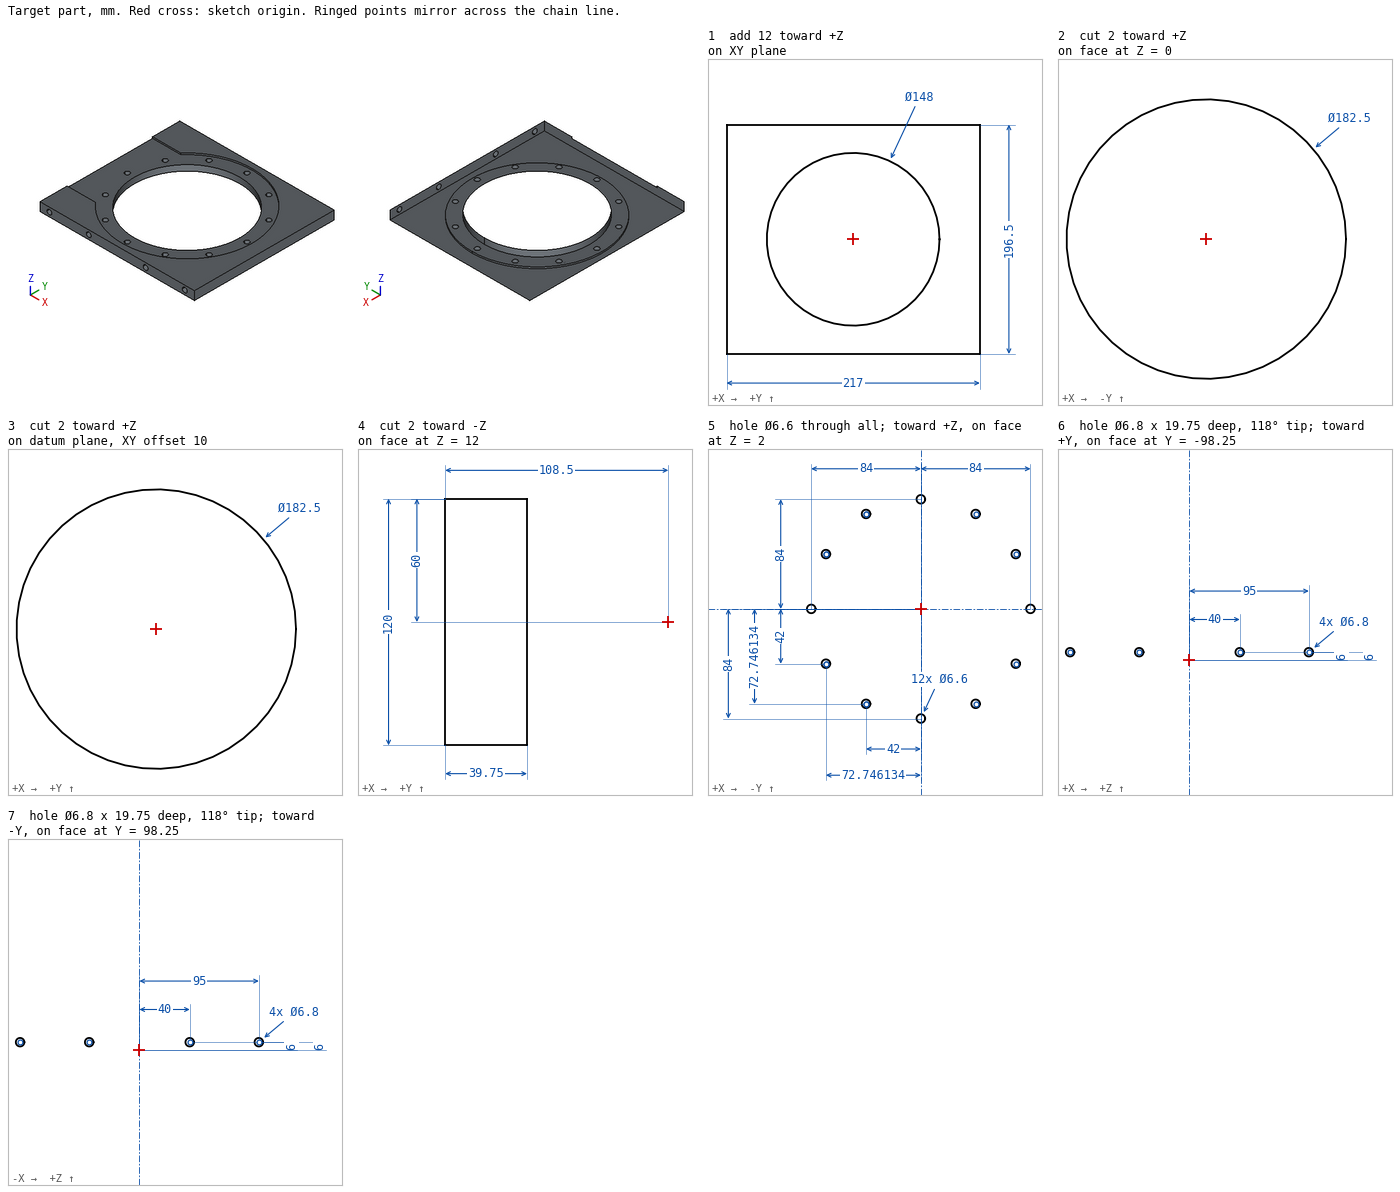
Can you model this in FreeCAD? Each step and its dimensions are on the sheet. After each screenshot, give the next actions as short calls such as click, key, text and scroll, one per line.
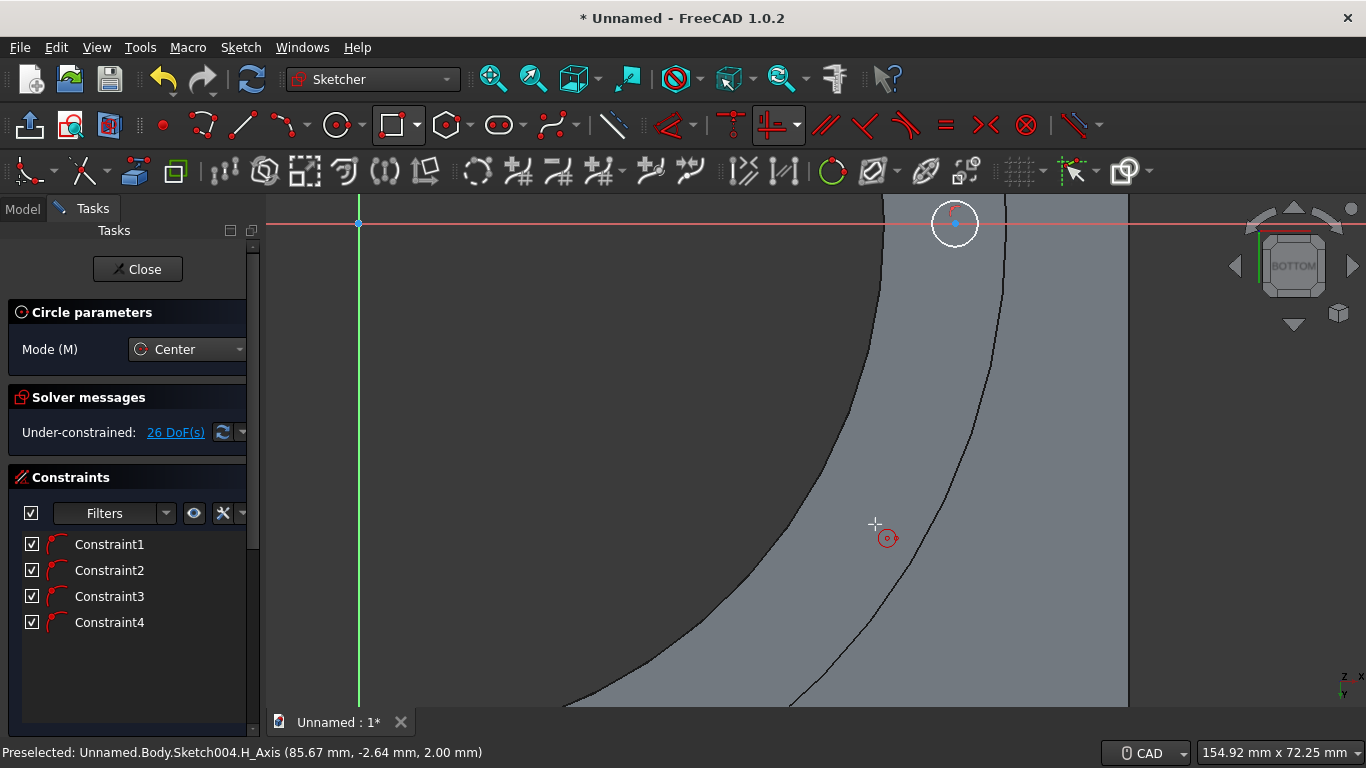
scroll(875, 525, down, 7)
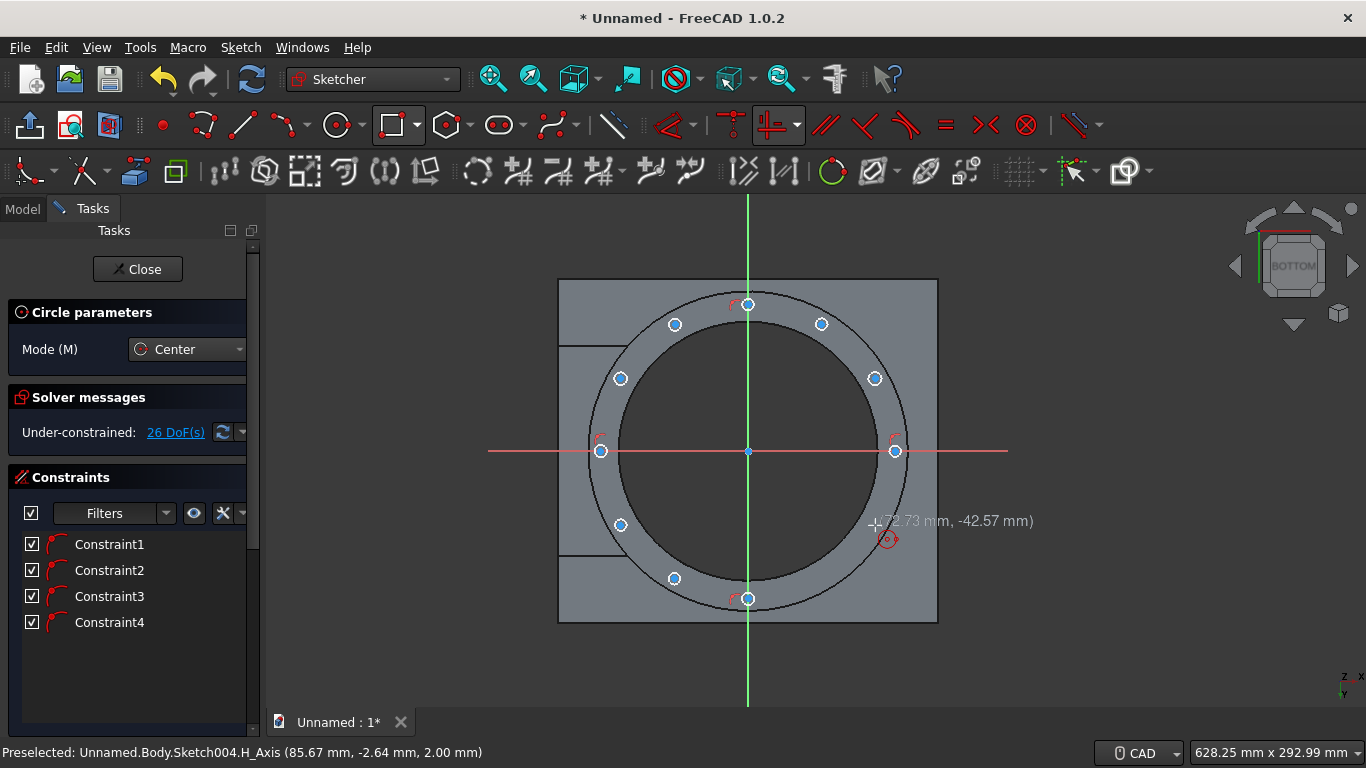
click(875, 525)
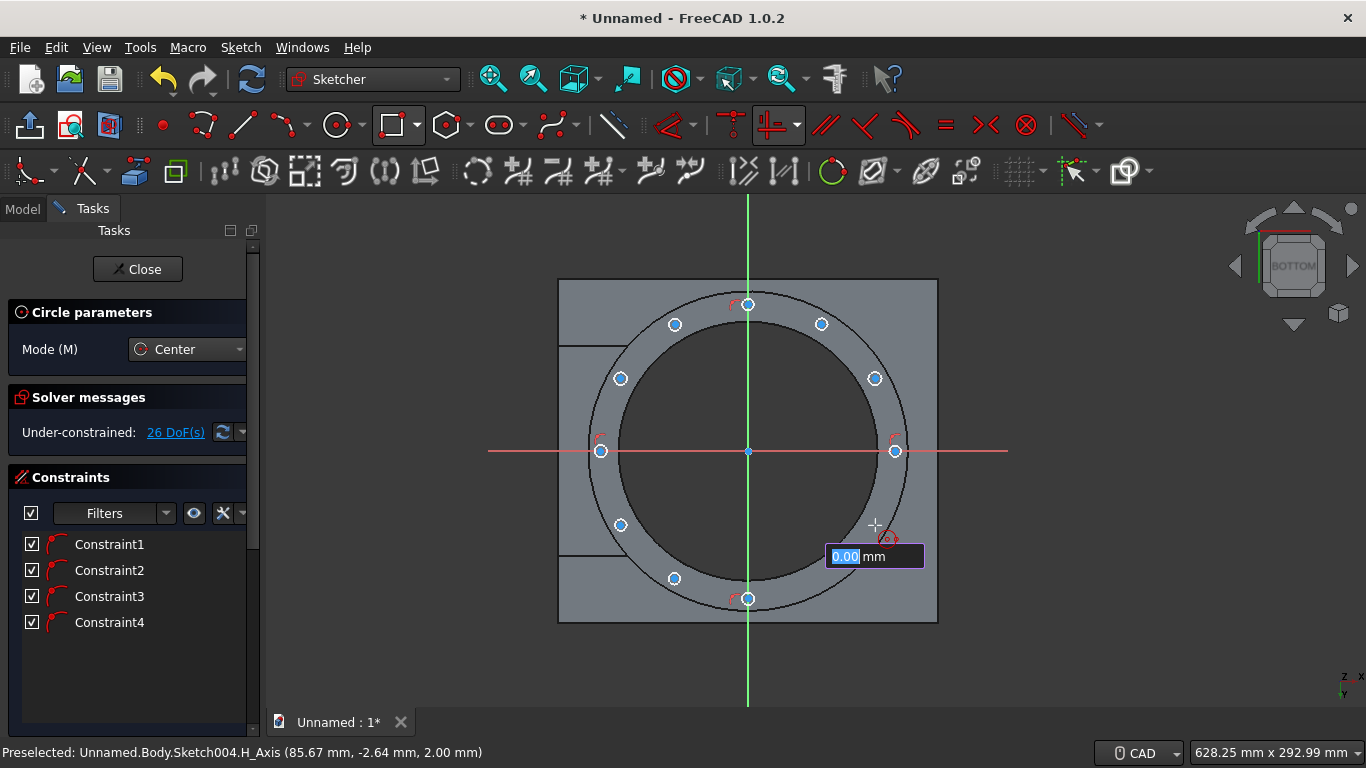
scroll(880, 521, up, 6)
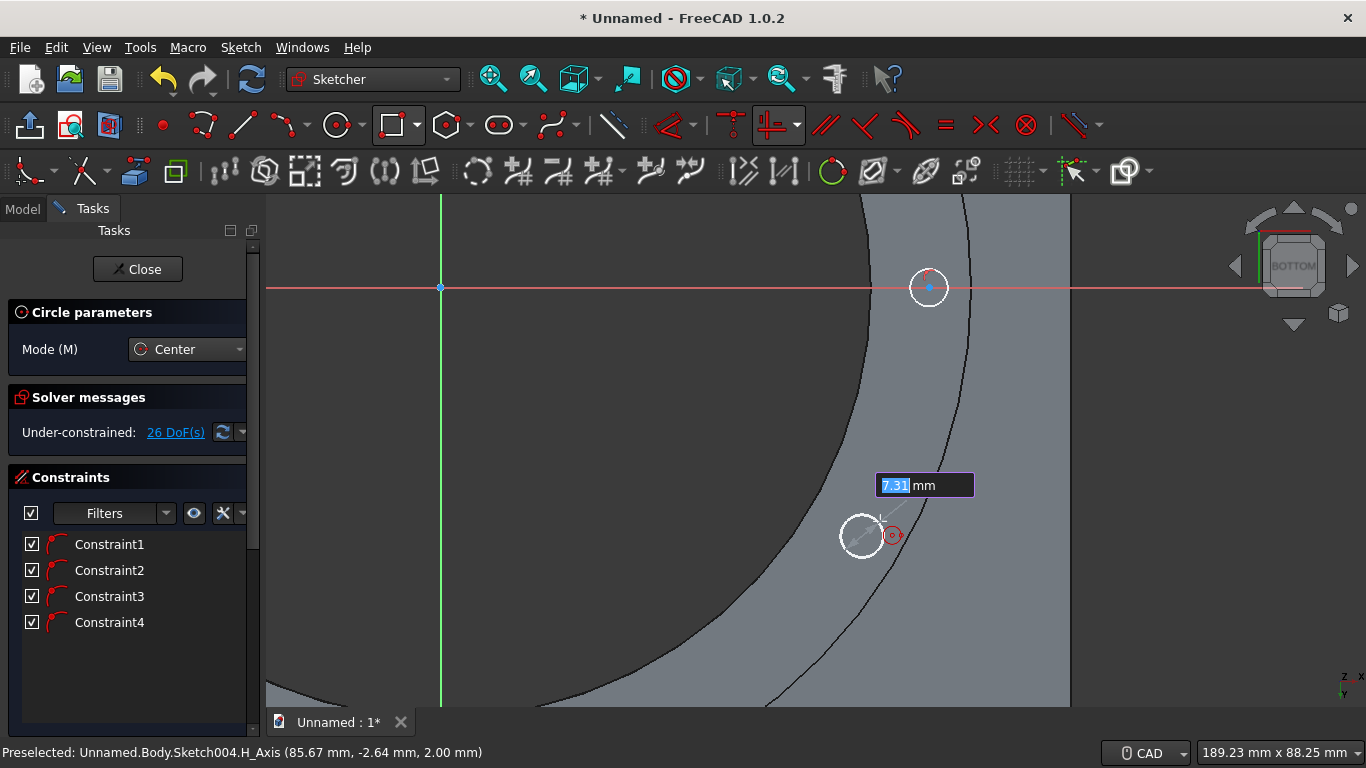
click(877, 518)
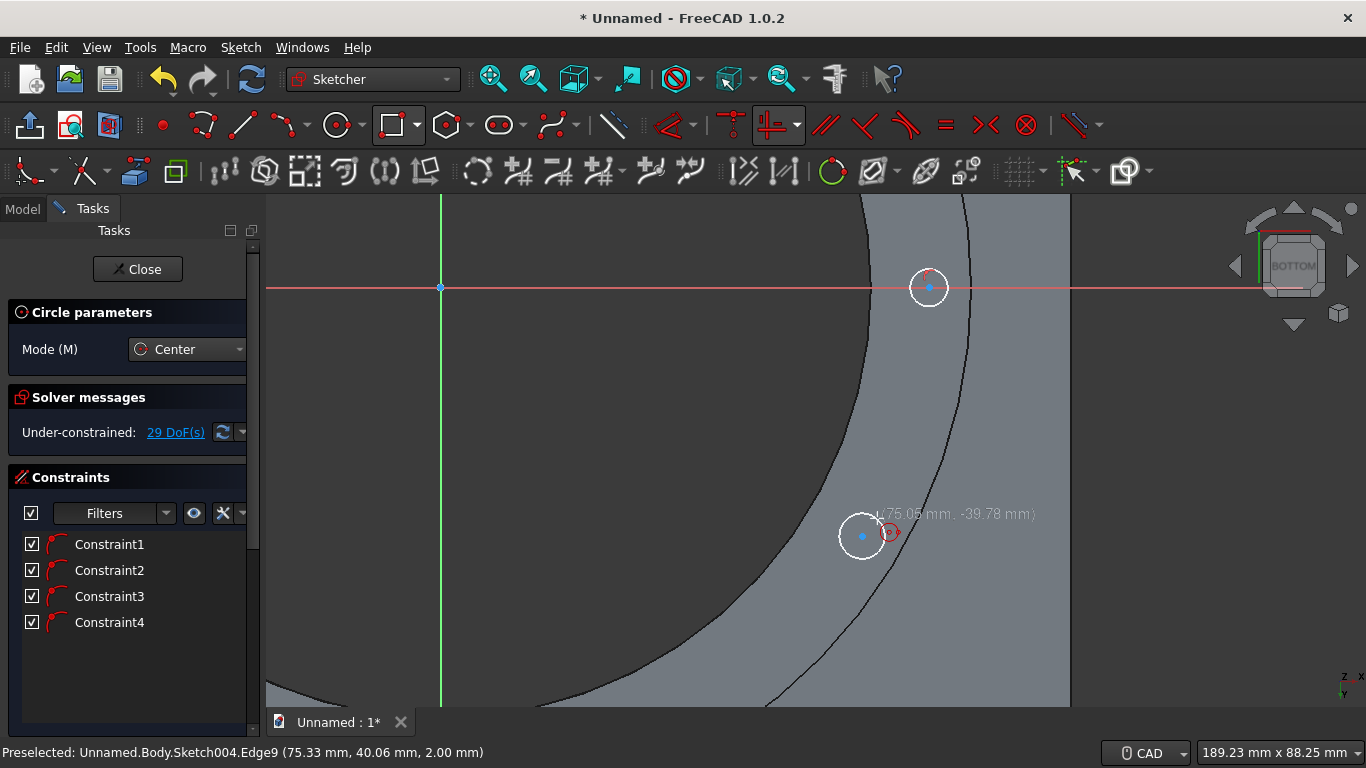
scroll(880, 521, down, 6)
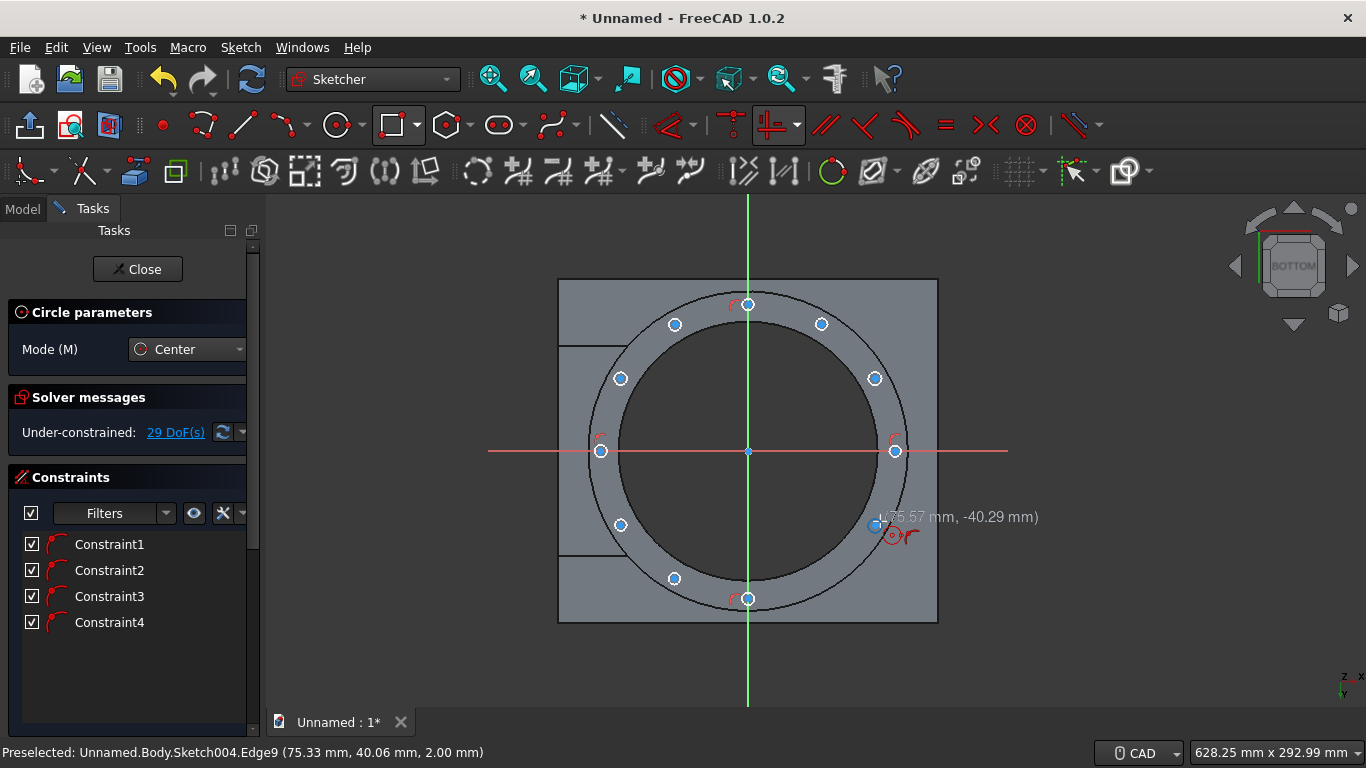
scroll(822, 579, up, 7)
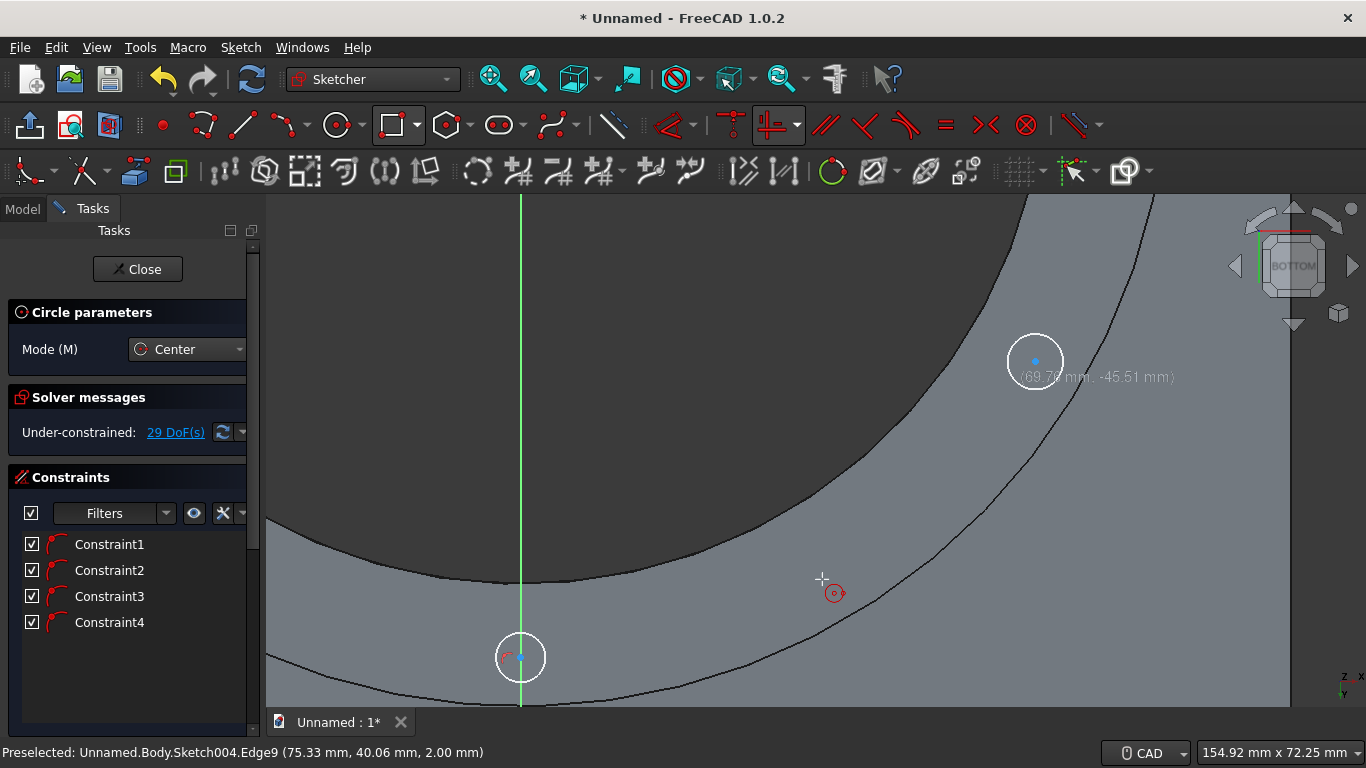
scroll(822, 579, down, 7)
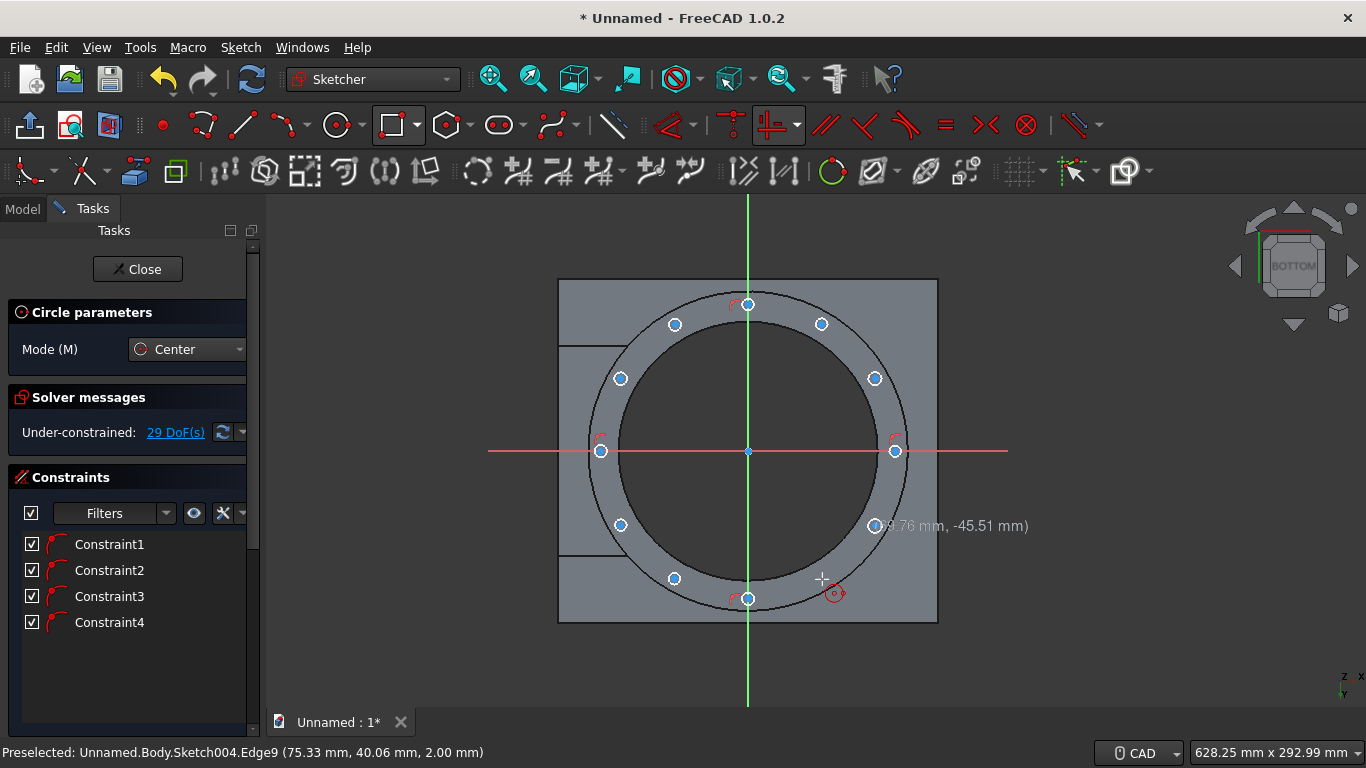
click(822, 579)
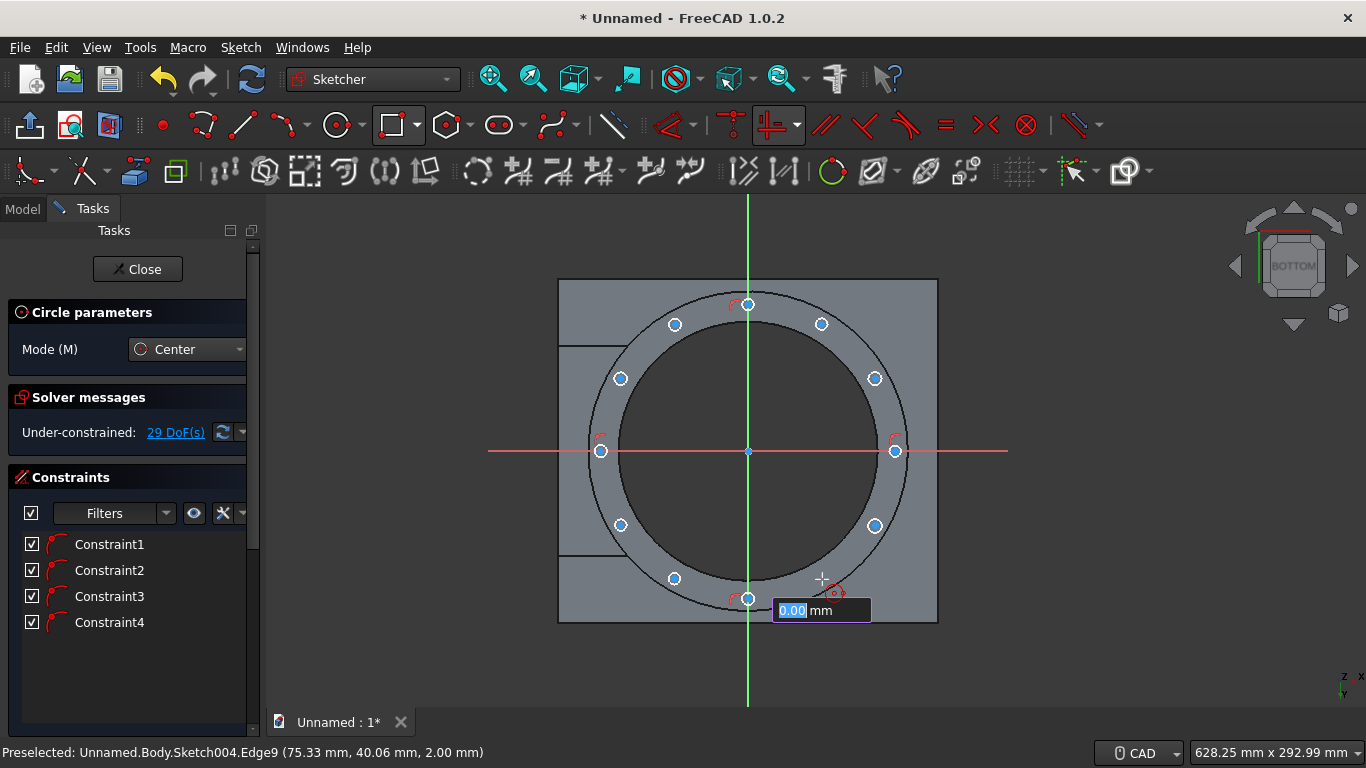
scroll(826, 574, up, 6)